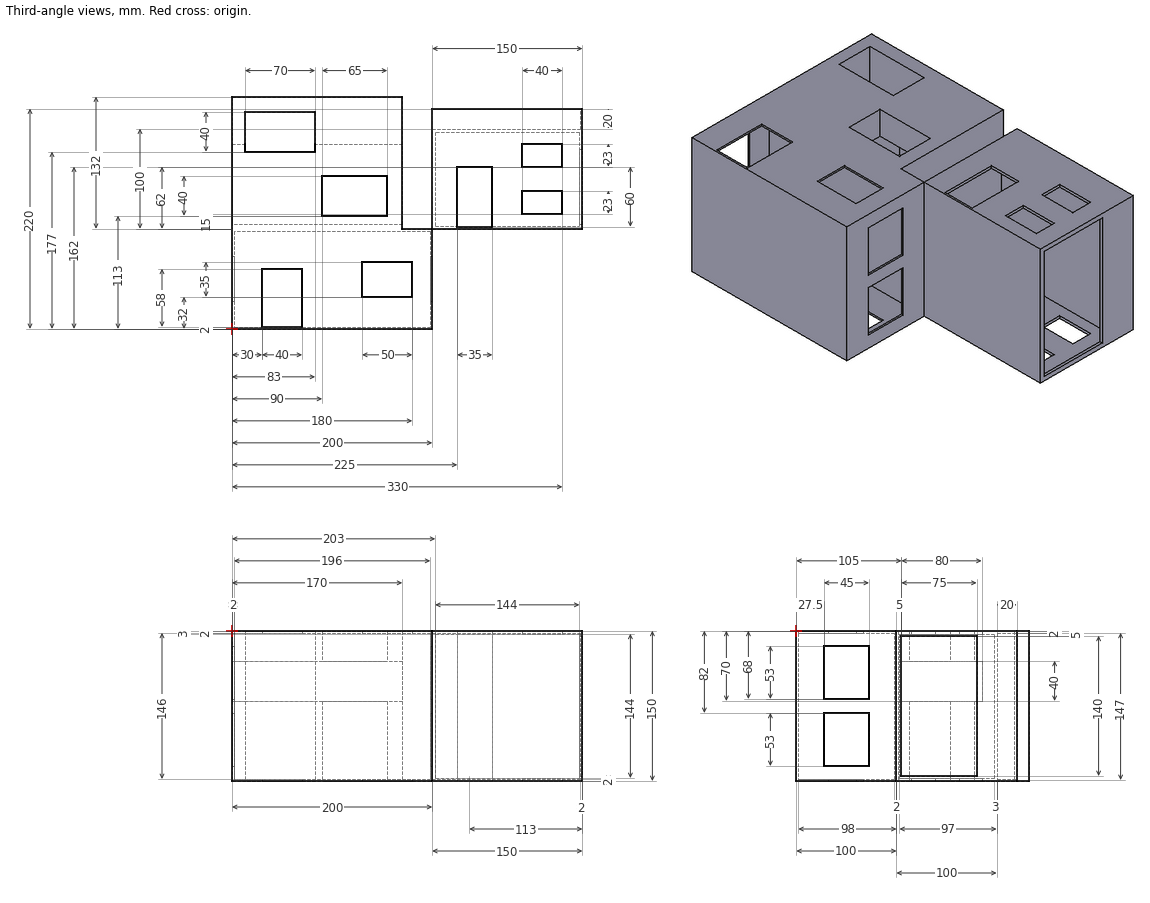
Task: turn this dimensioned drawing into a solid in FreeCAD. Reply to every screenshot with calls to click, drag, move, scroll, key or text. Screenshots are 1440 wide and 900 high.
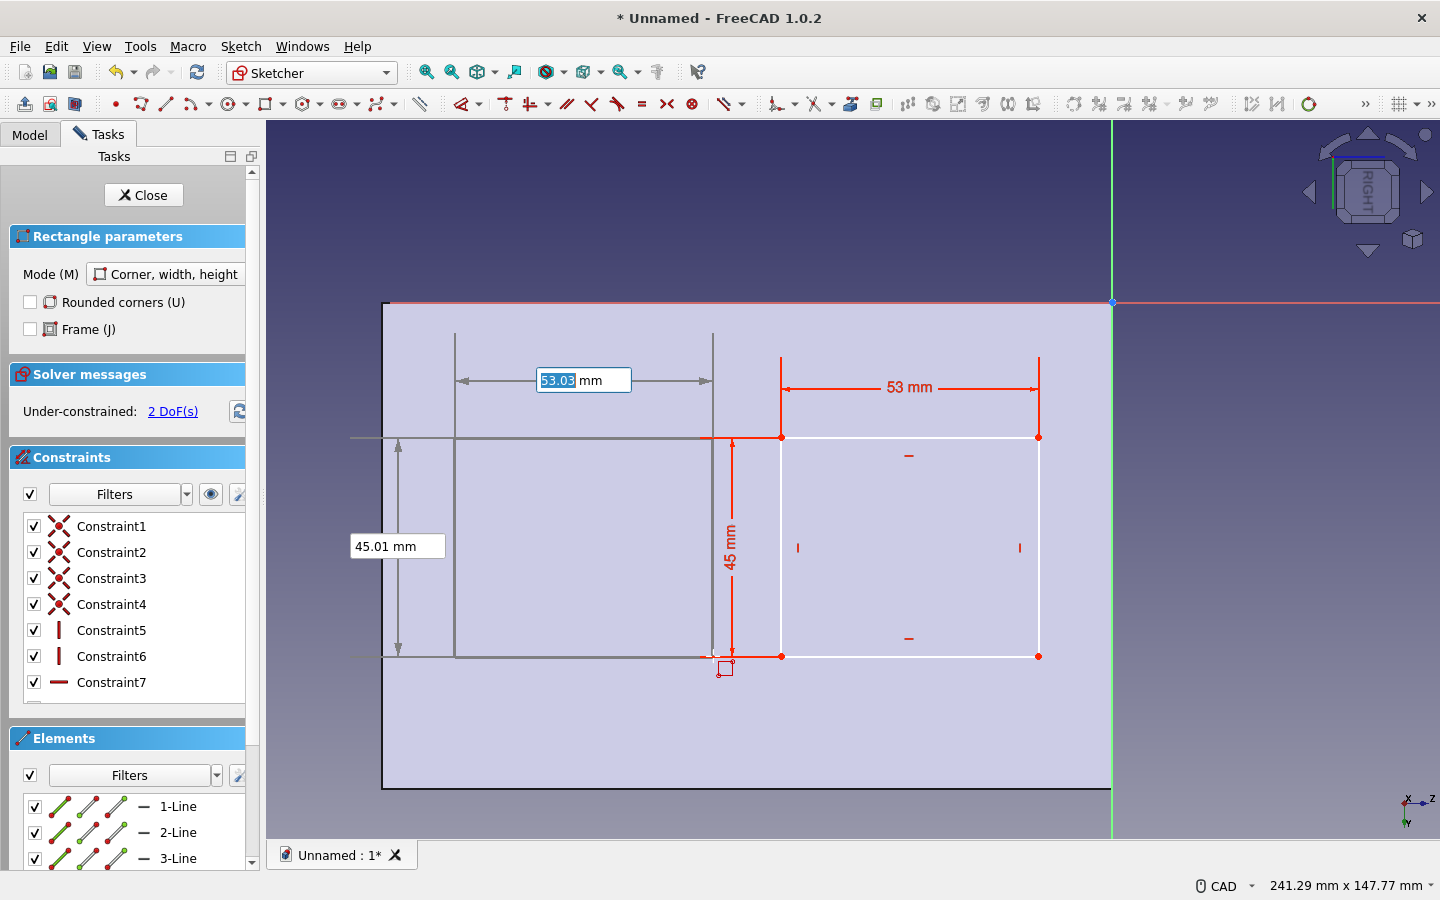
text(53)
key(Tab)
text(45)
key(Return)
key(Escape)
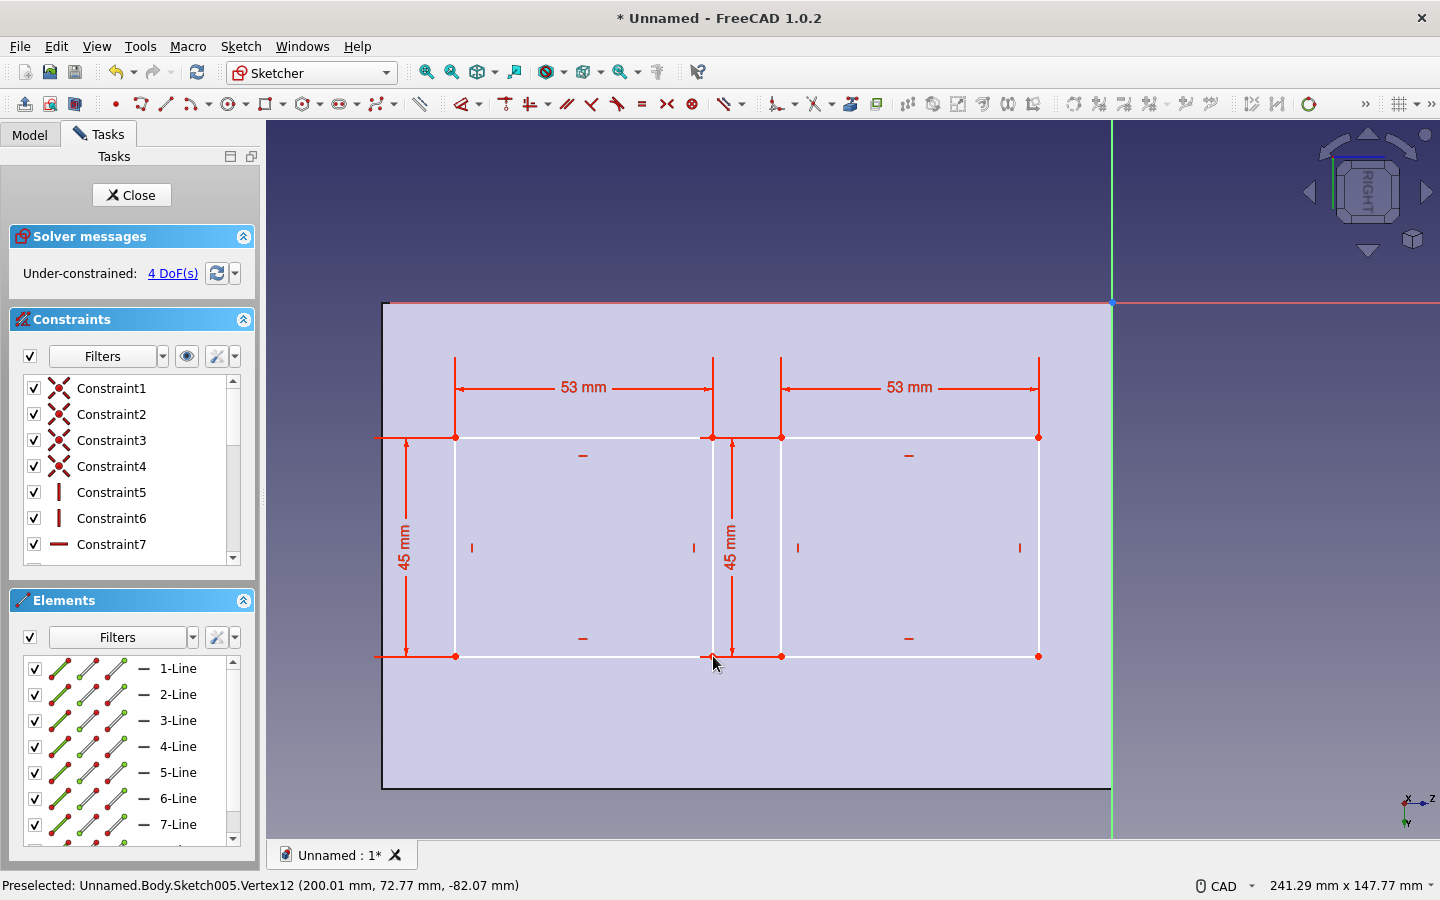
click(460, 104)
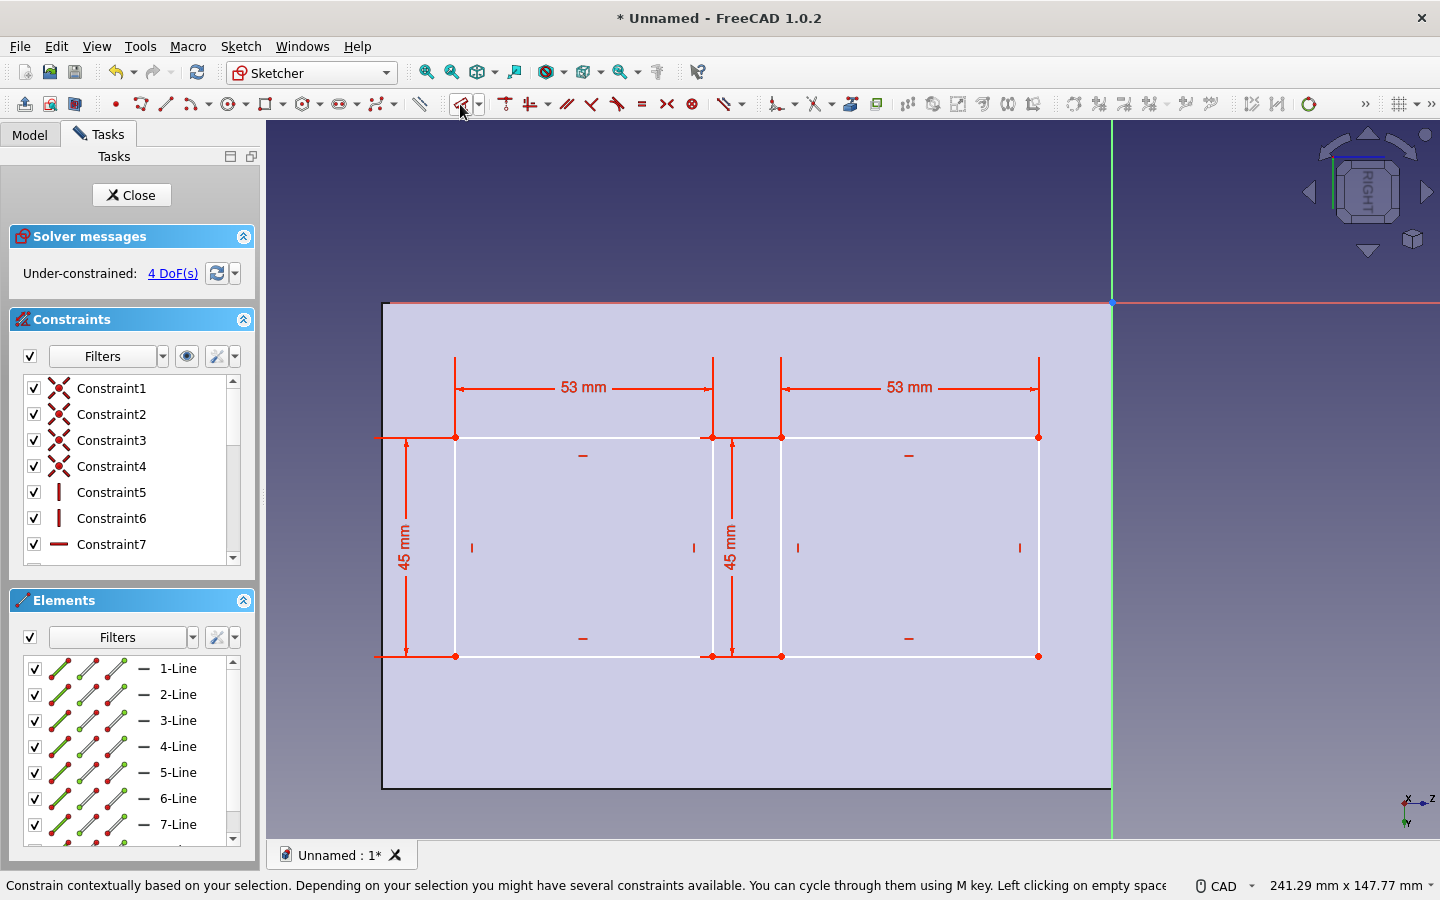
click(781, 438)
click(947, 269)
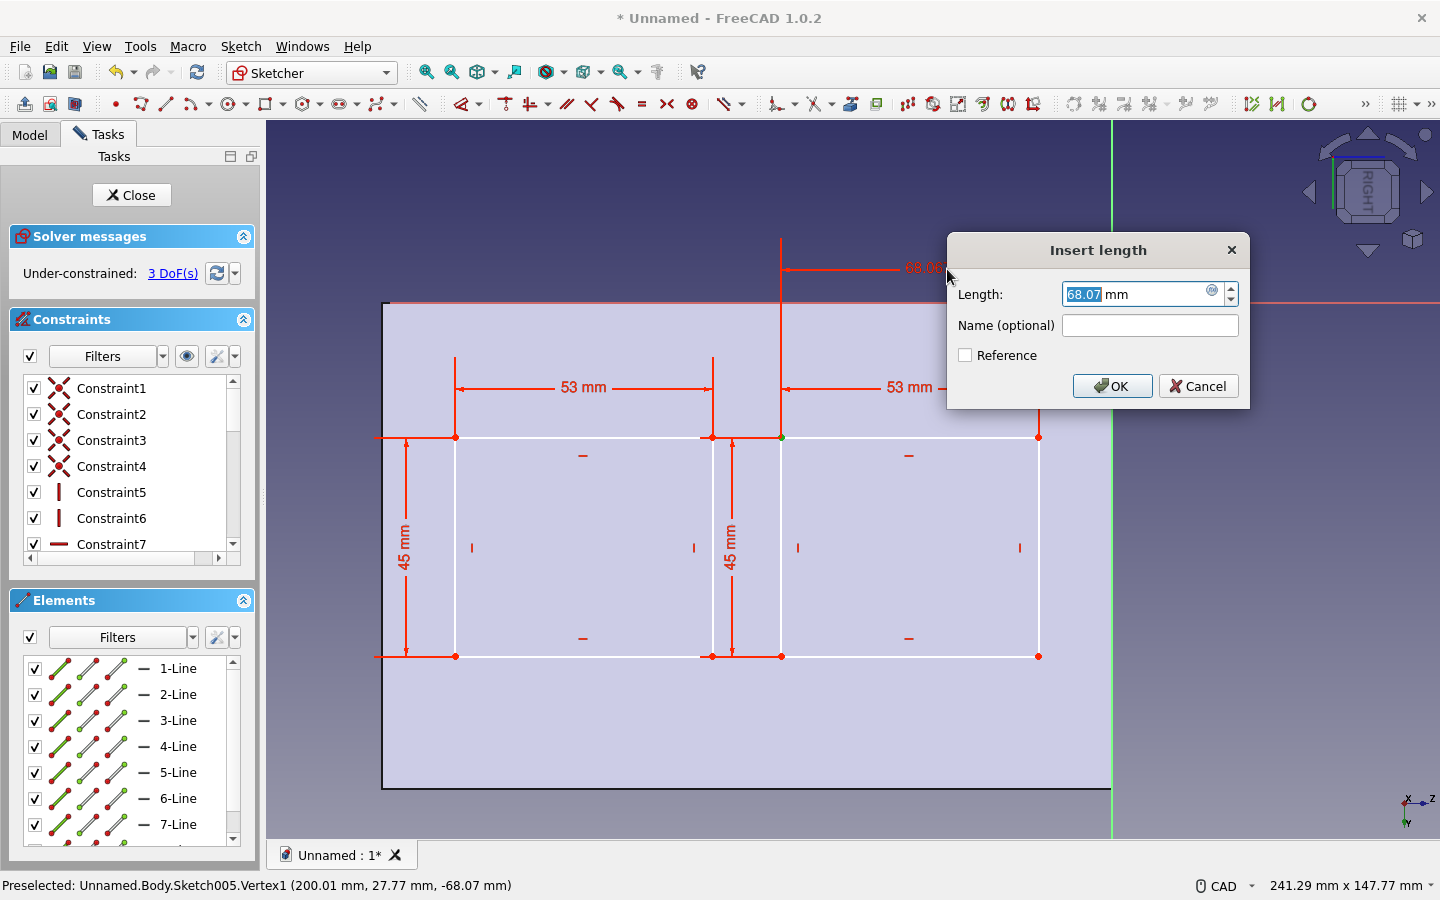
text(68)
key(Return)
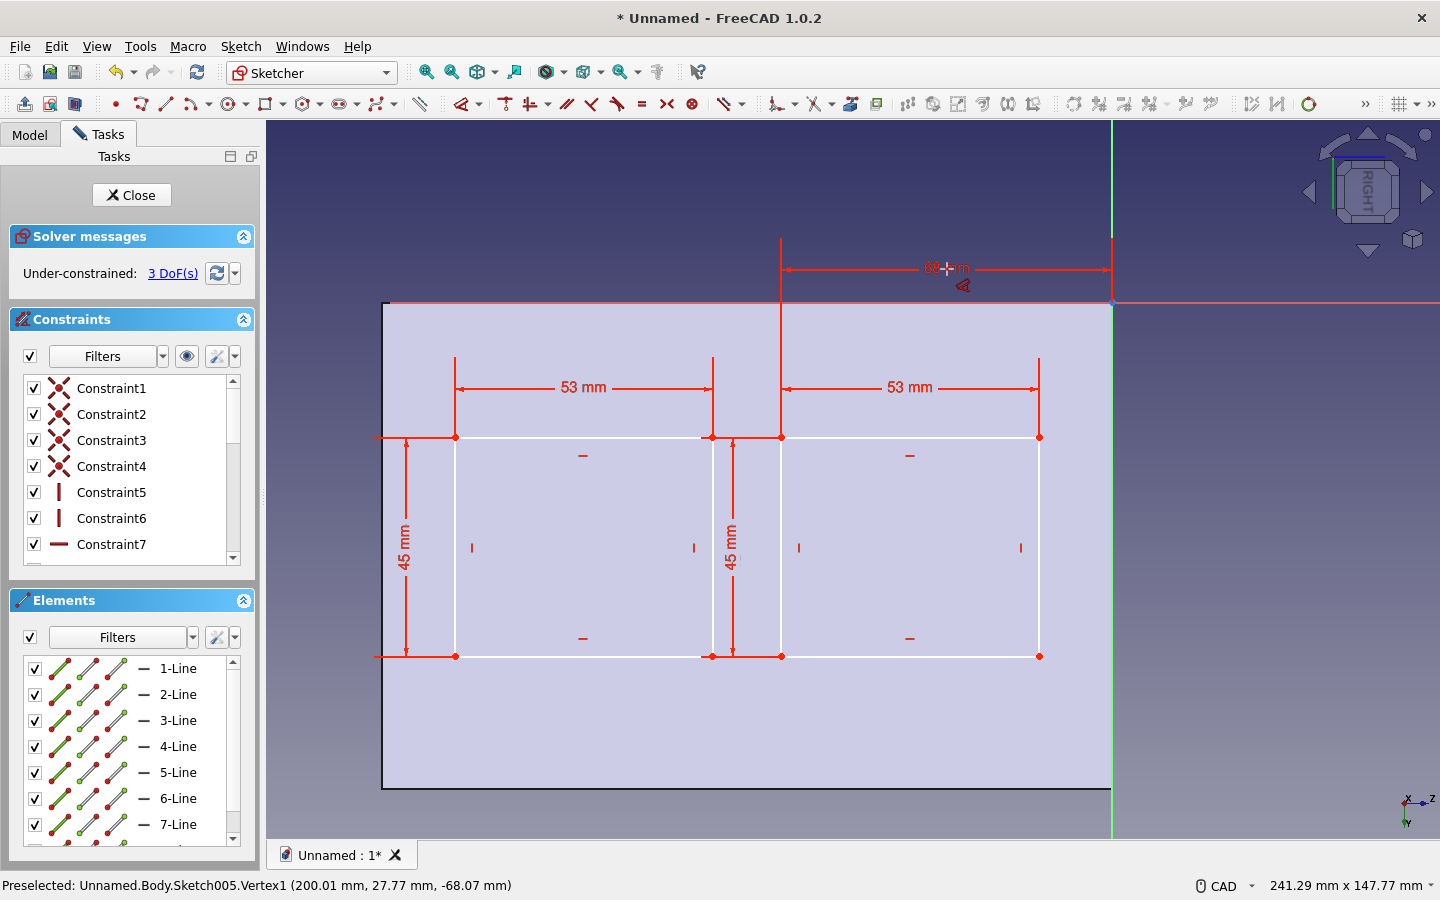
click(713, 657)
click(913, 691)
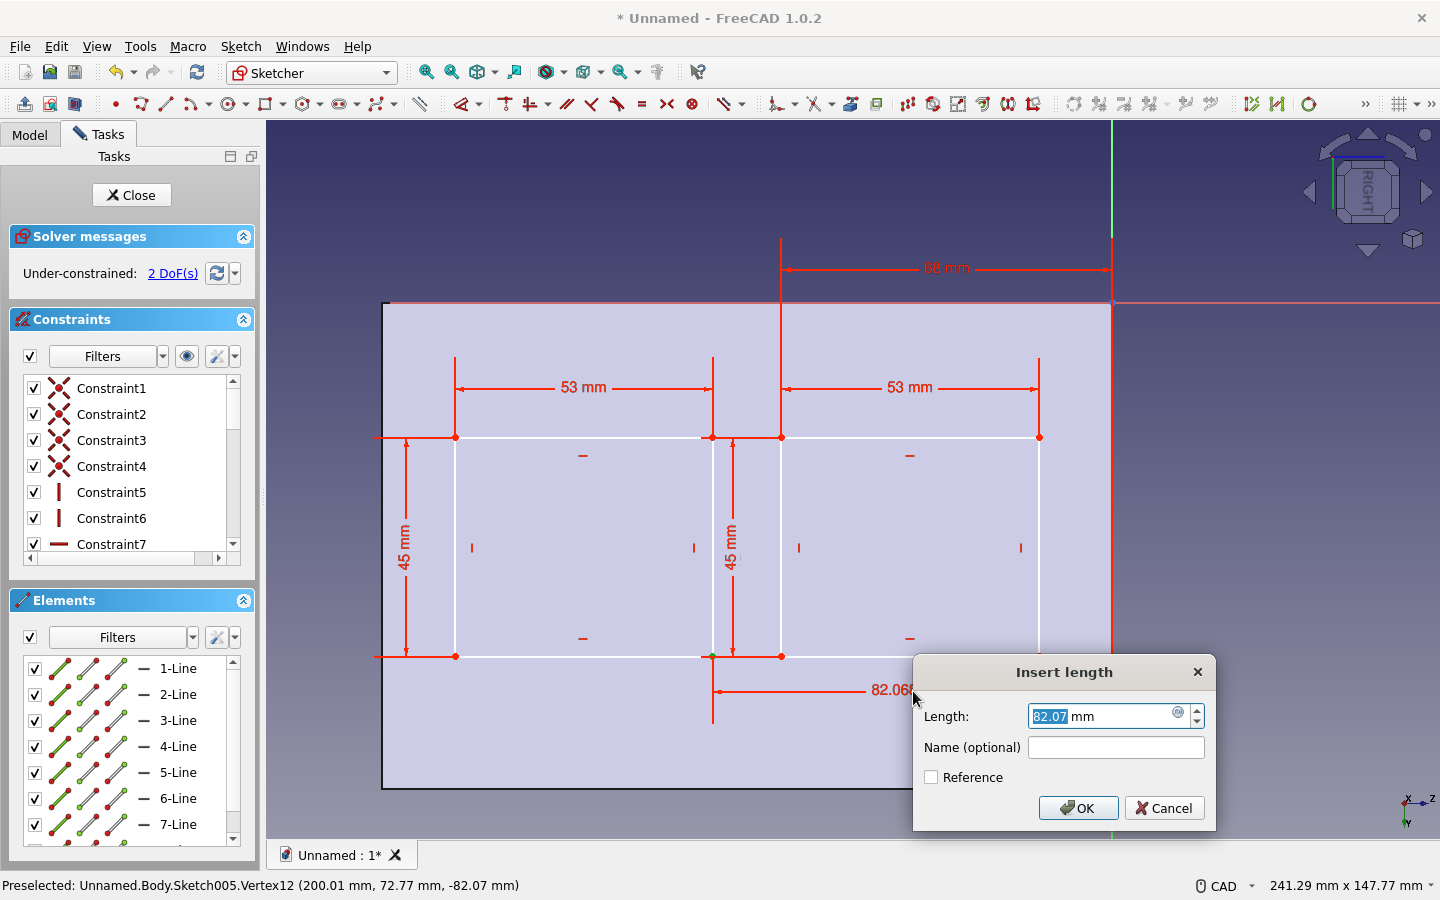
text(82)
key(Return)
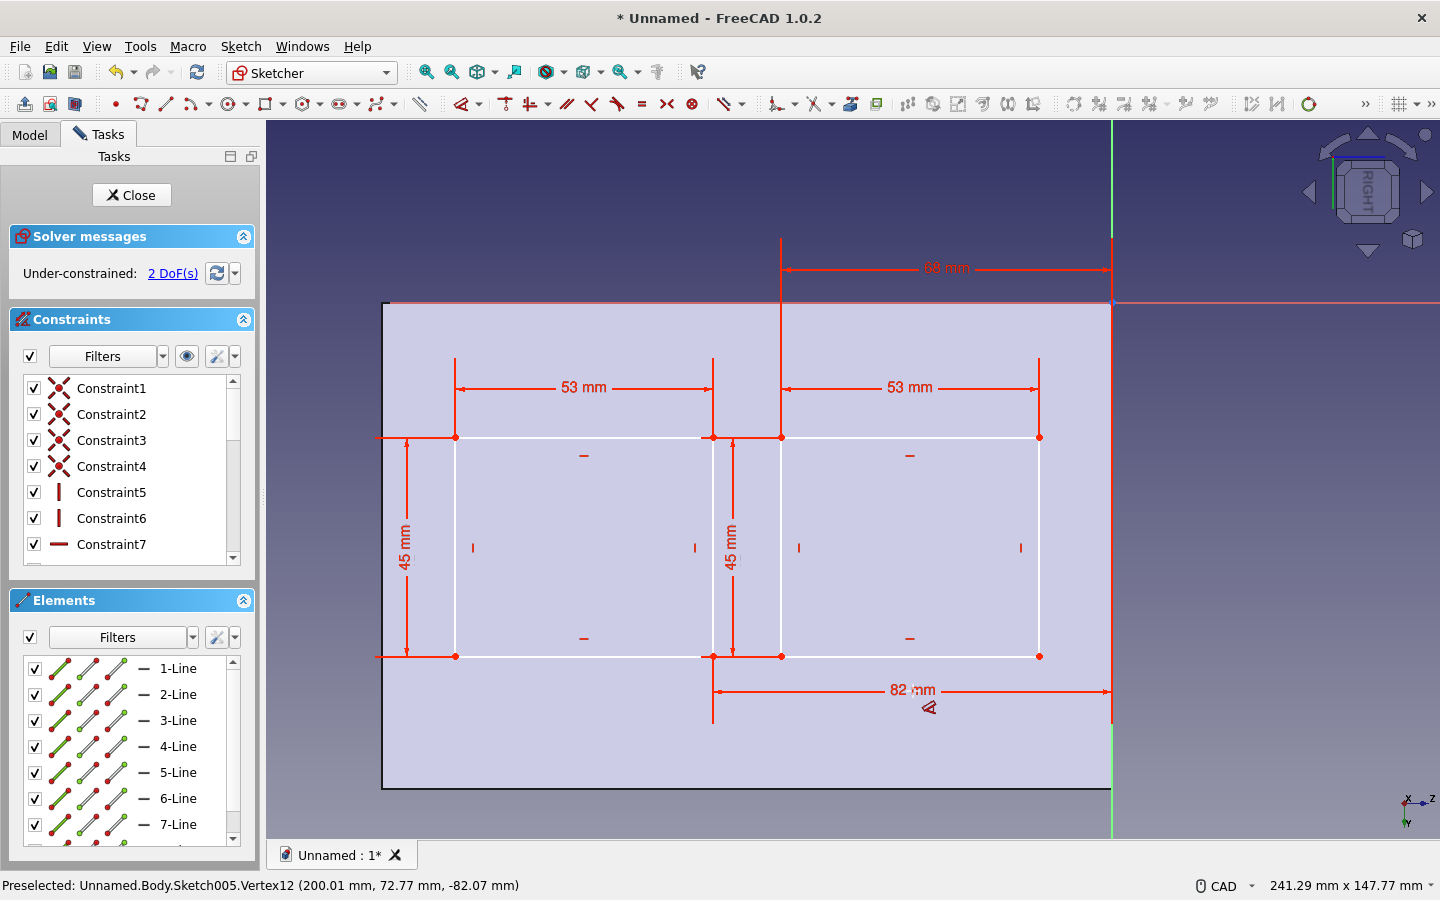
click(781, 438)
click(1146, 370)